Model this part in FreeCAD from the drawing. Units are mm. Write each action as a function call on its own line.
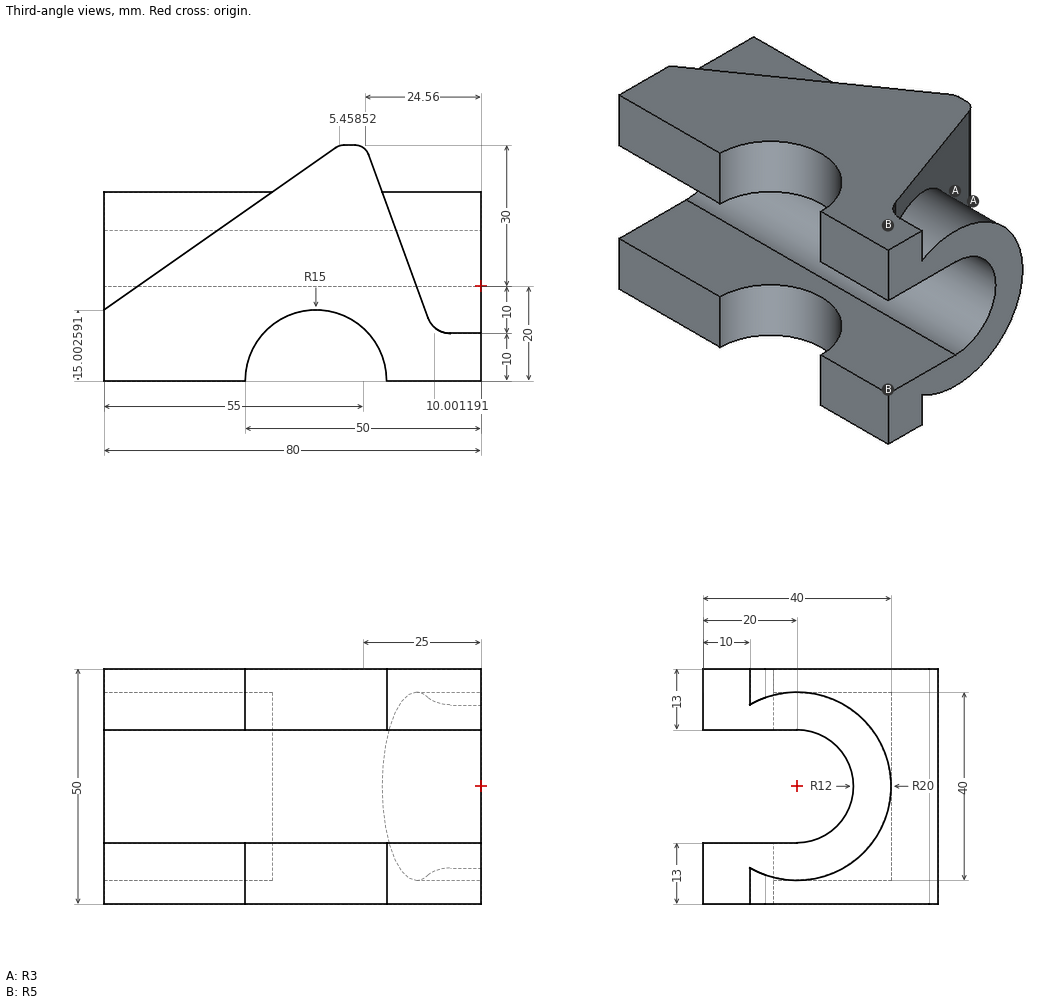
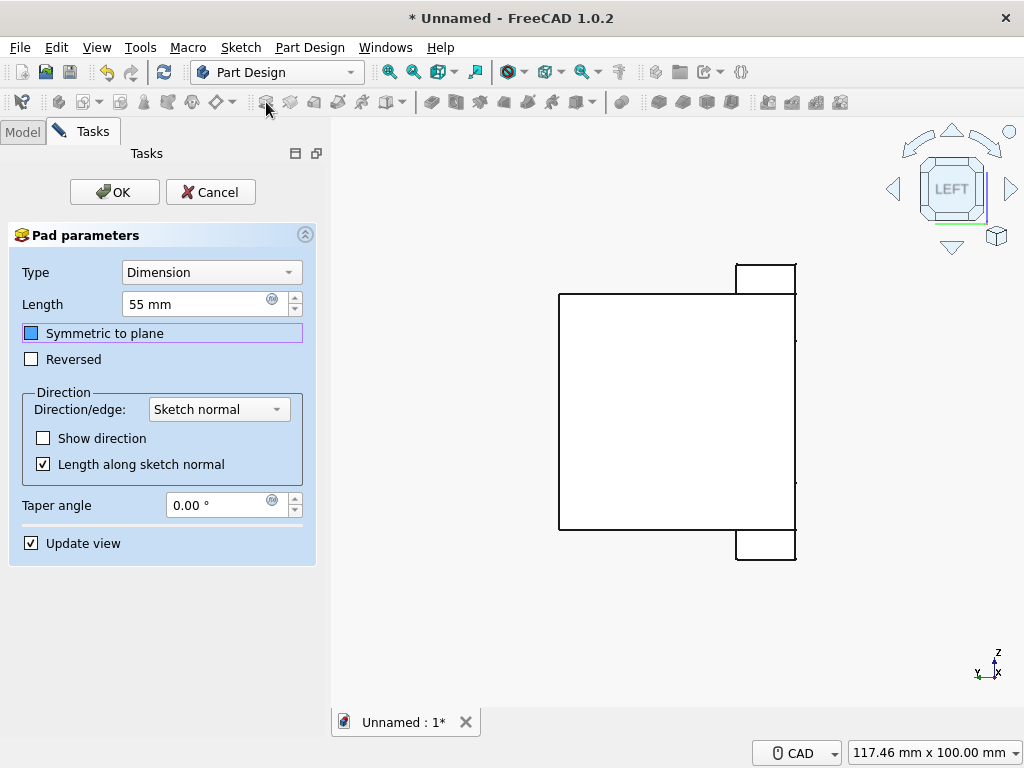
click(115, 192)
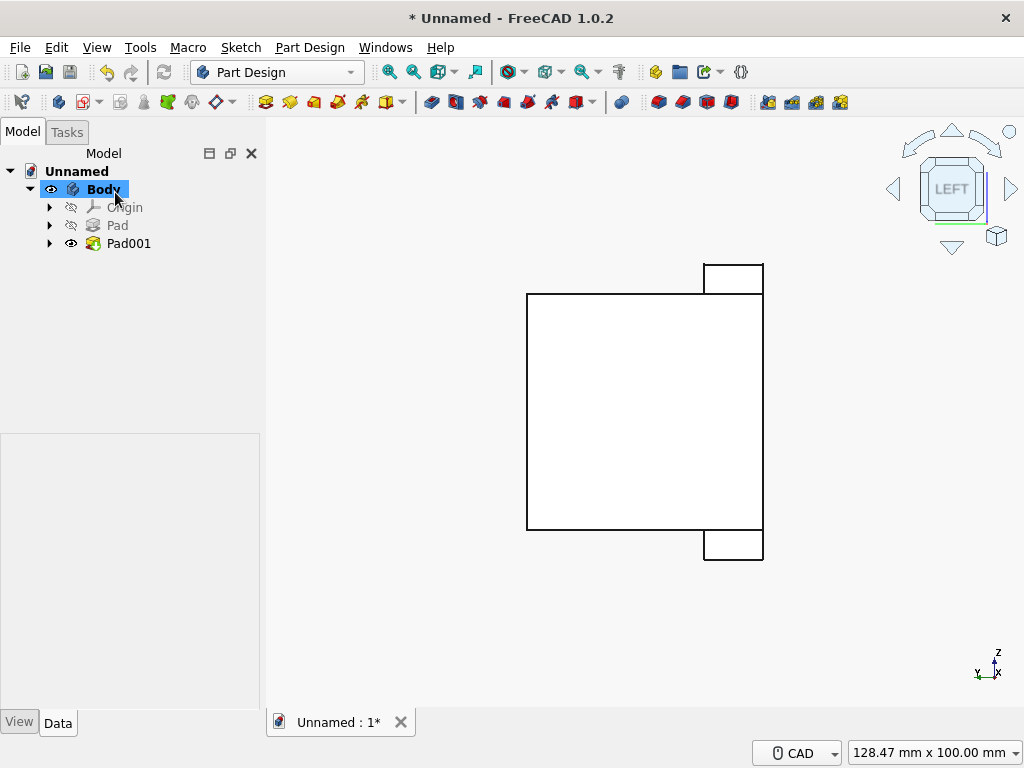
click(84, 102)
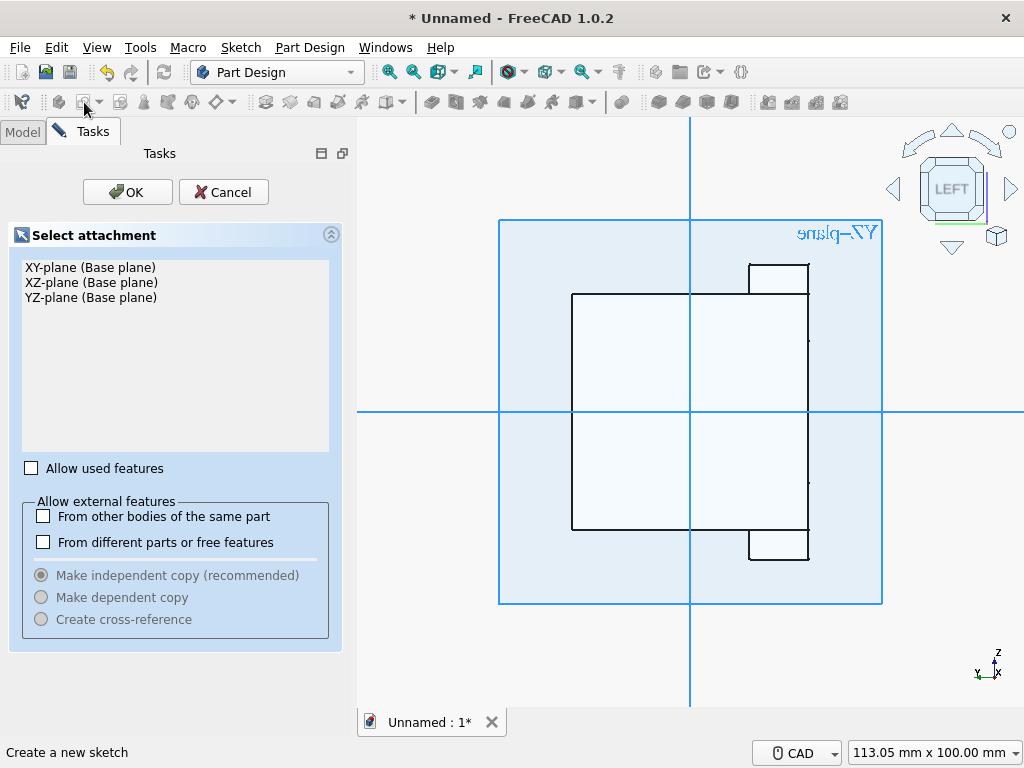
click(82, 268)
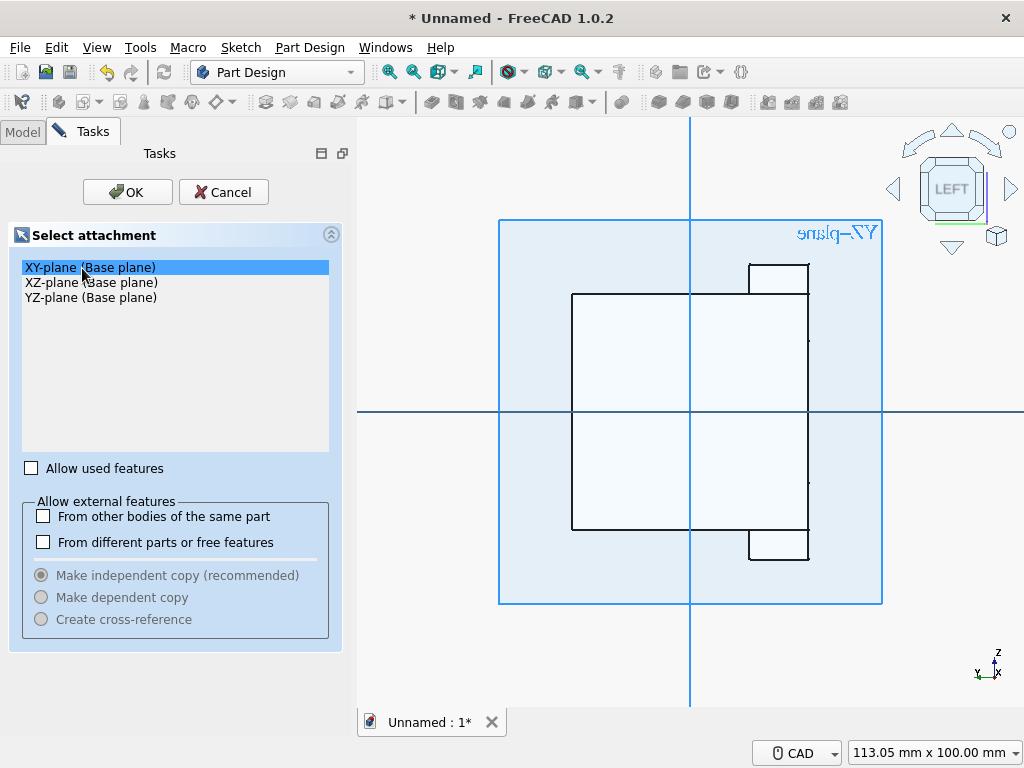
click(128, 192)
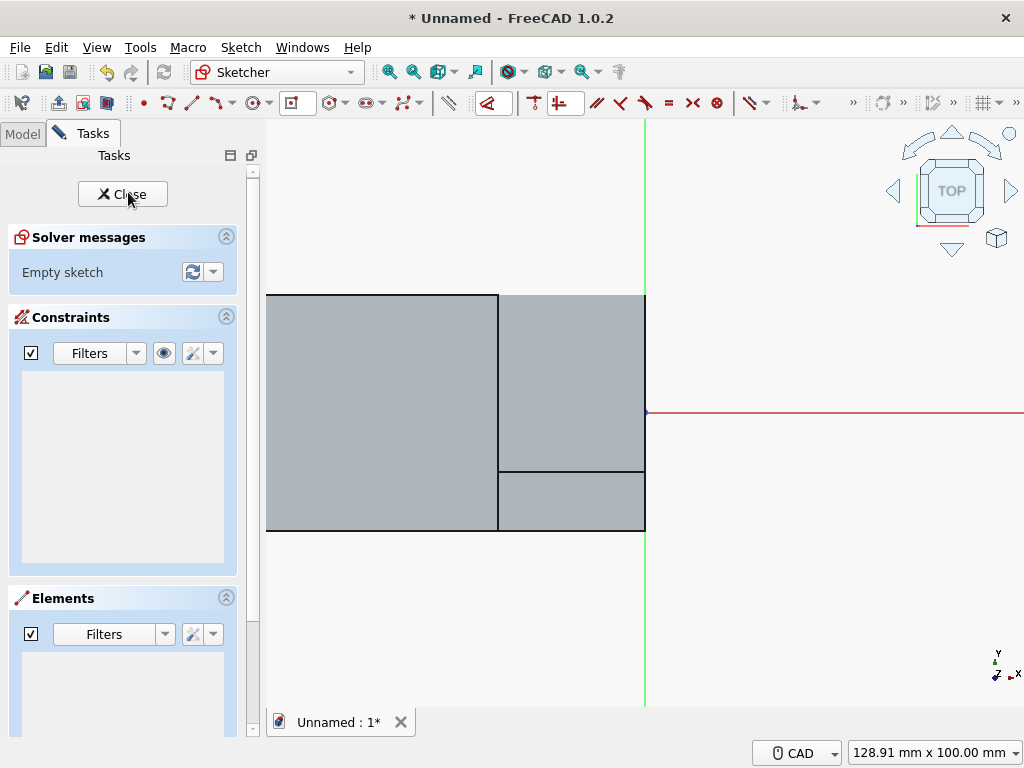
click(108, 104)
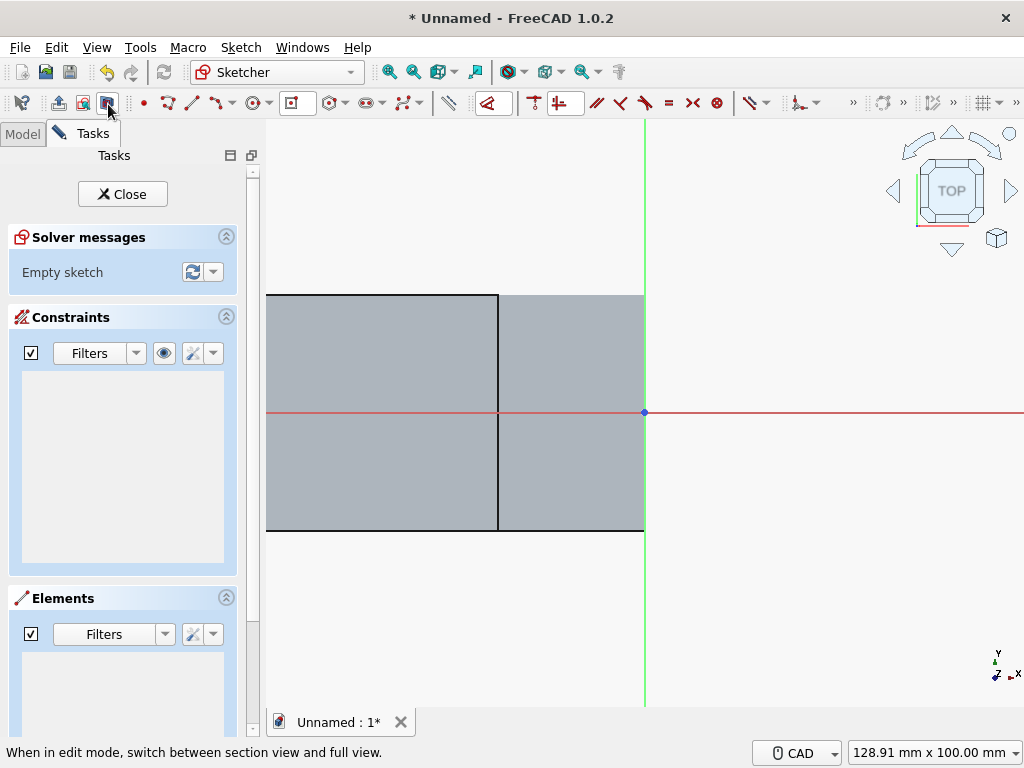
scroll(859, 473, down, 2)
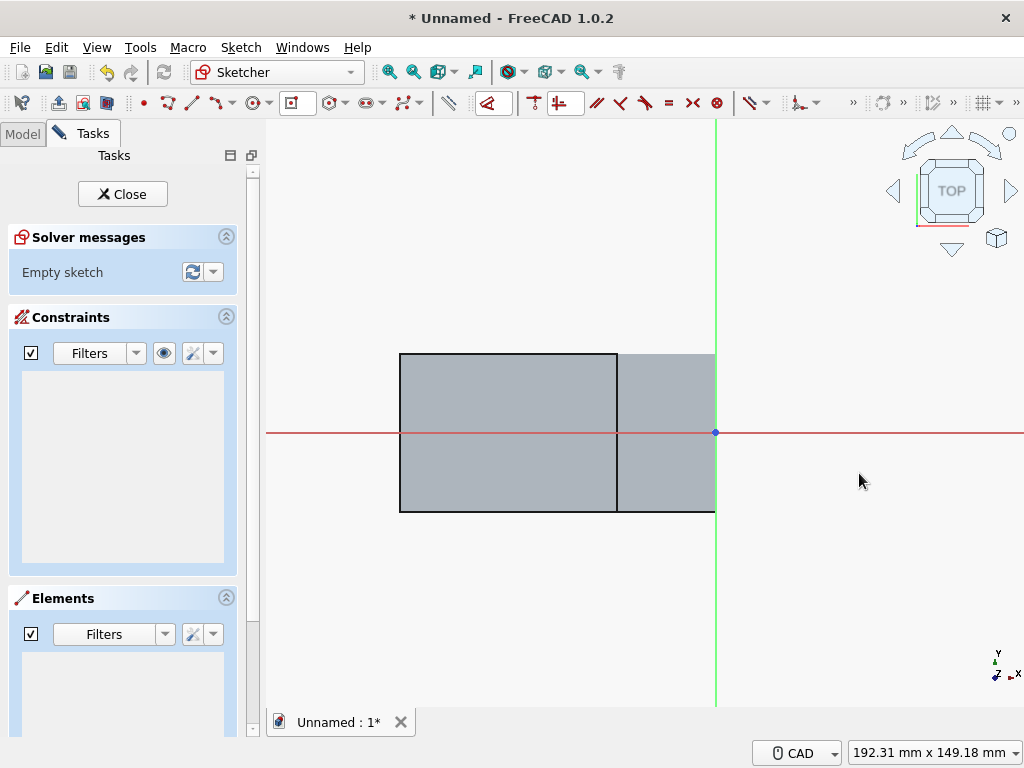
key(g)
key(m)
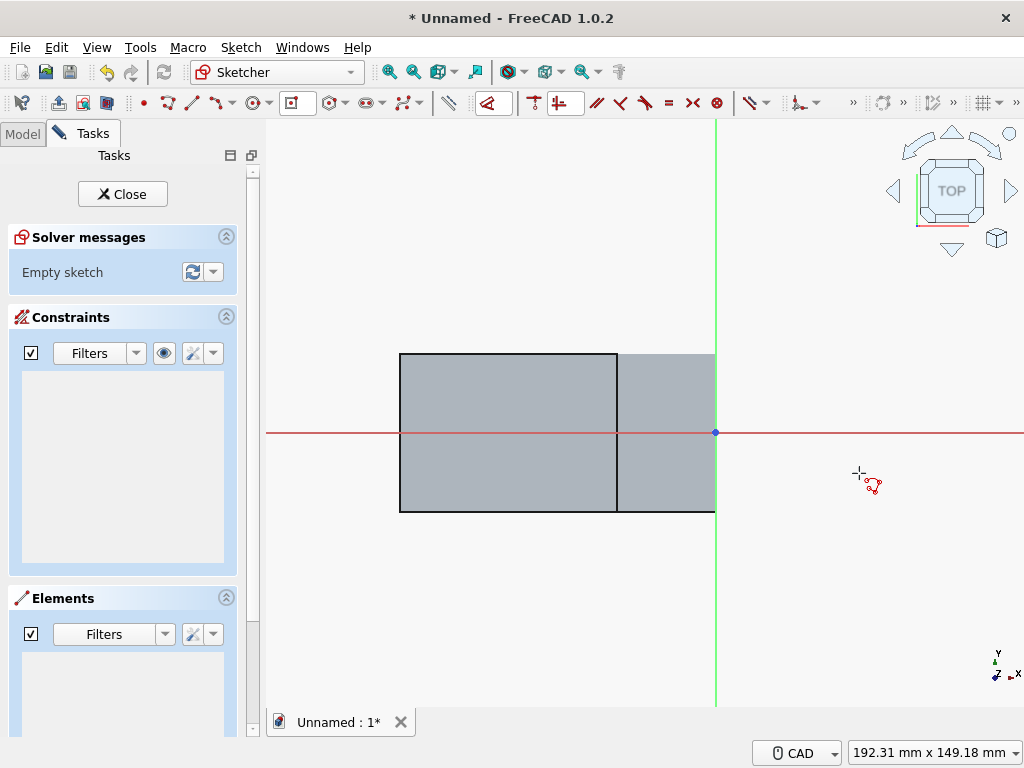
click(716, 472)
click(676, 472)
click(619, 315)
click(597, 315)
click(400, 453)
click(400, 512)
click(707, 512)
click(716, 473)
key(Escape)
key(Escape)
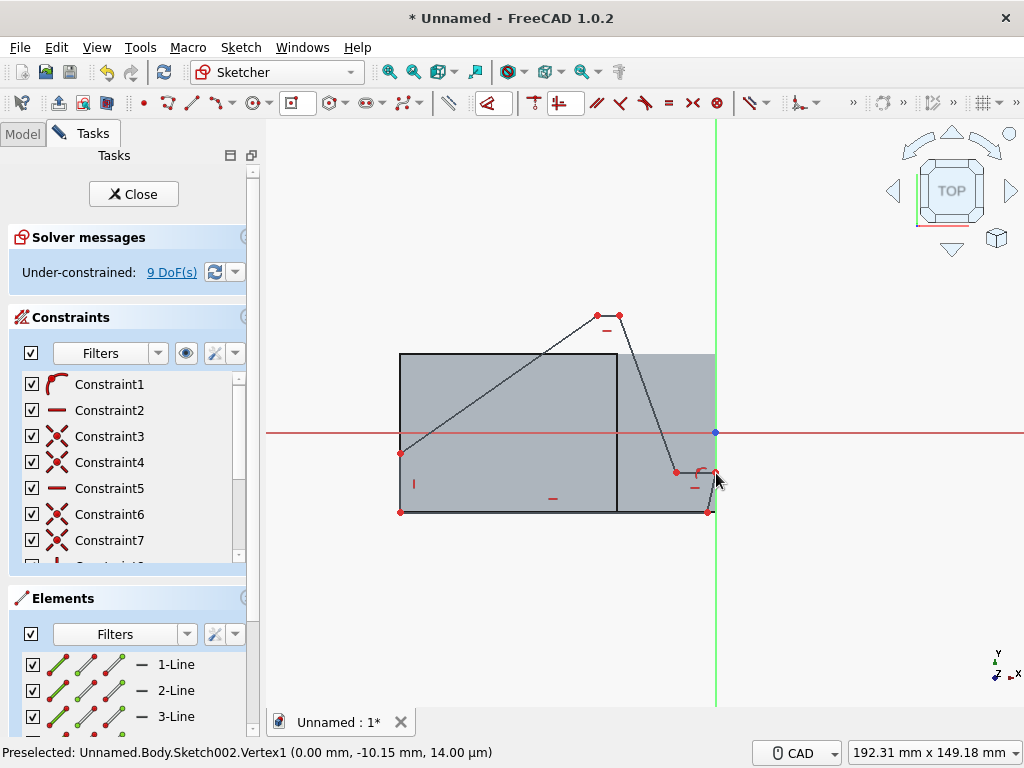
click(713, 485)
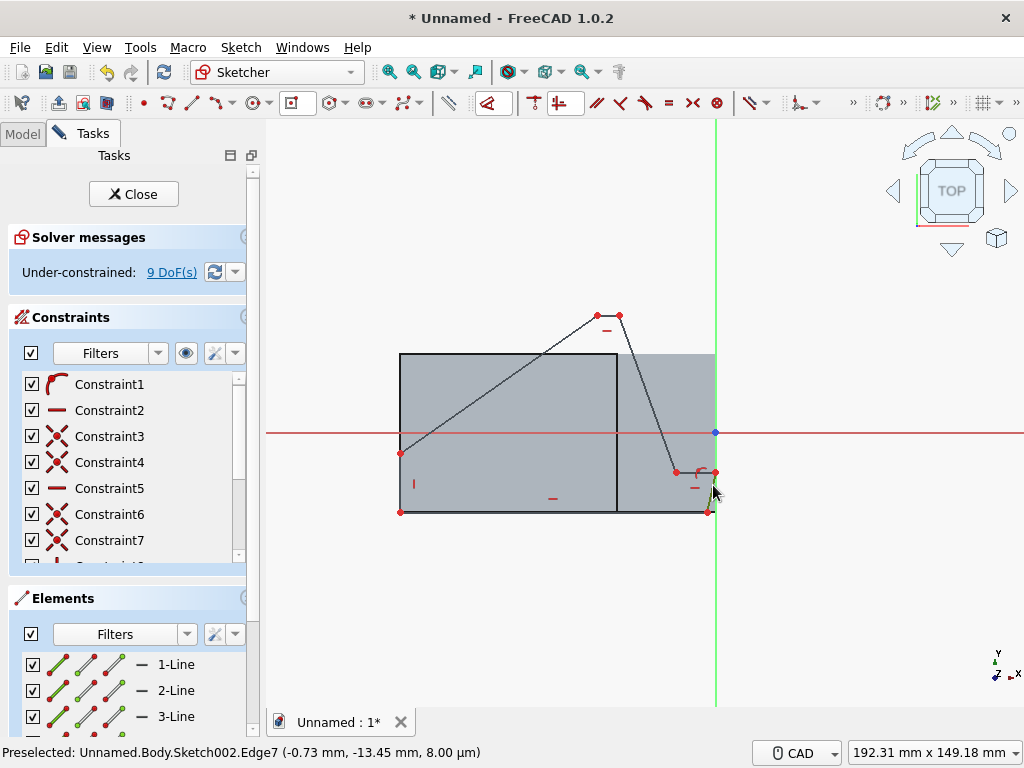
key(v)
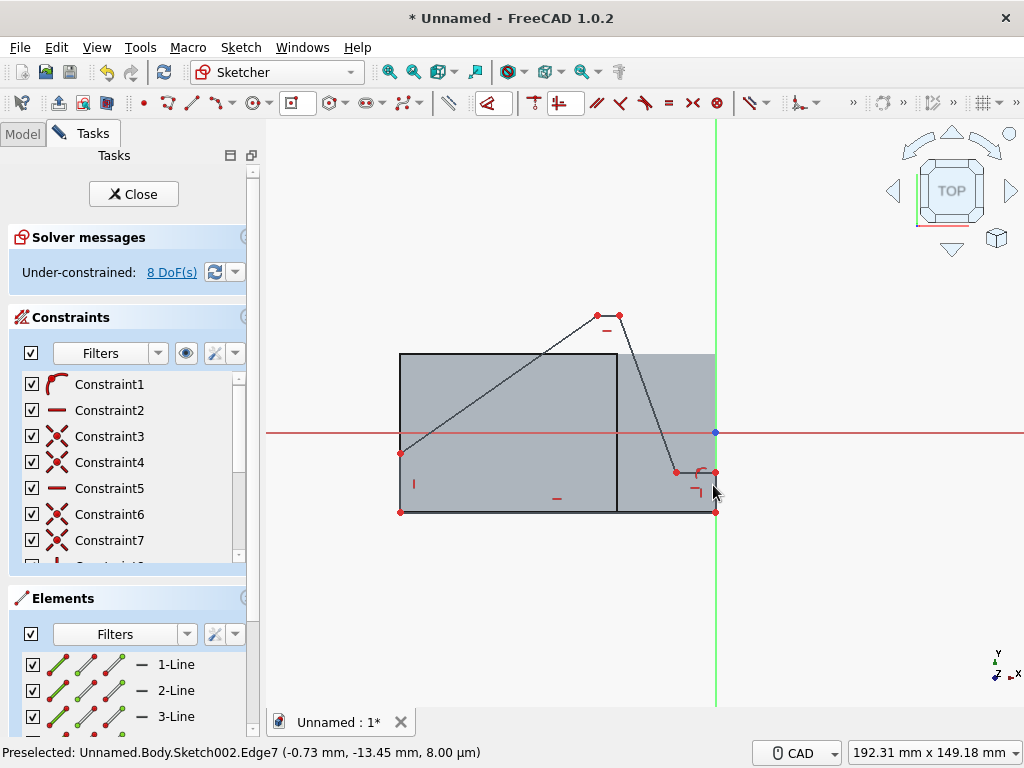
click(488, 104)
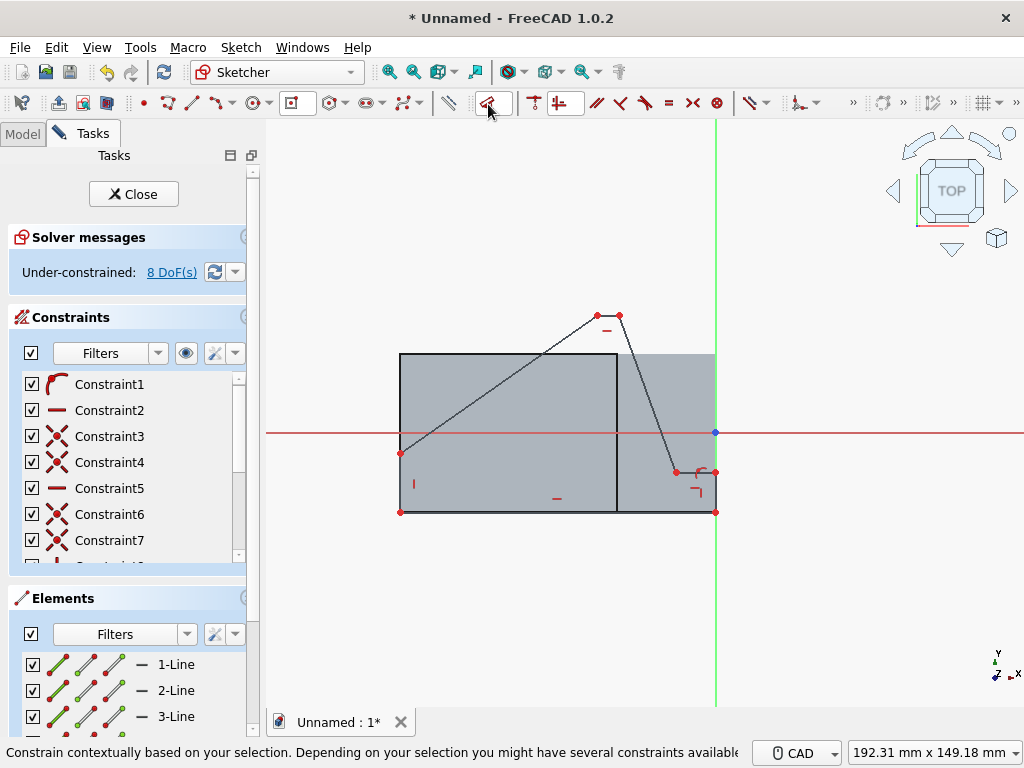
click(495, 513)
click(558, 547)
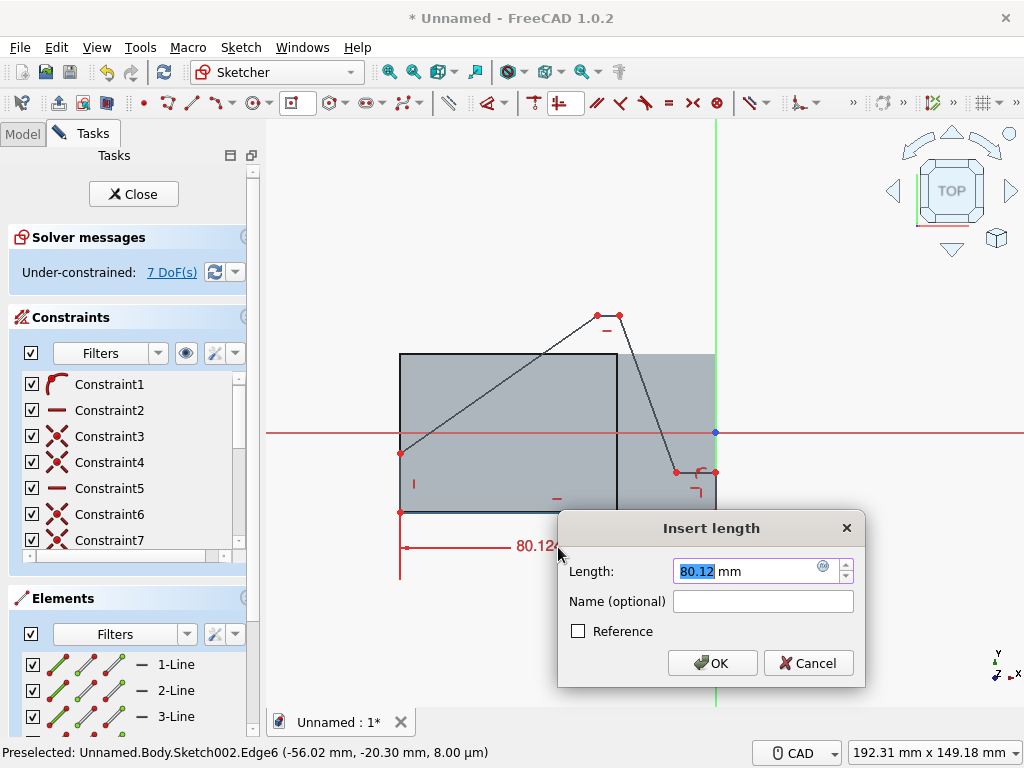
text(80)
key(Return)